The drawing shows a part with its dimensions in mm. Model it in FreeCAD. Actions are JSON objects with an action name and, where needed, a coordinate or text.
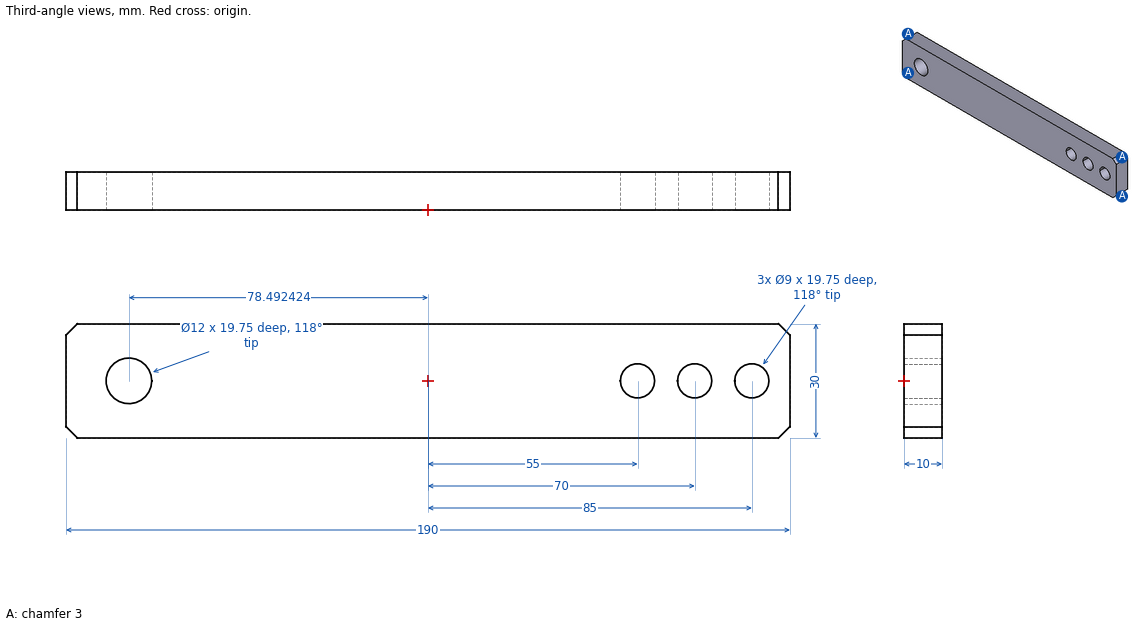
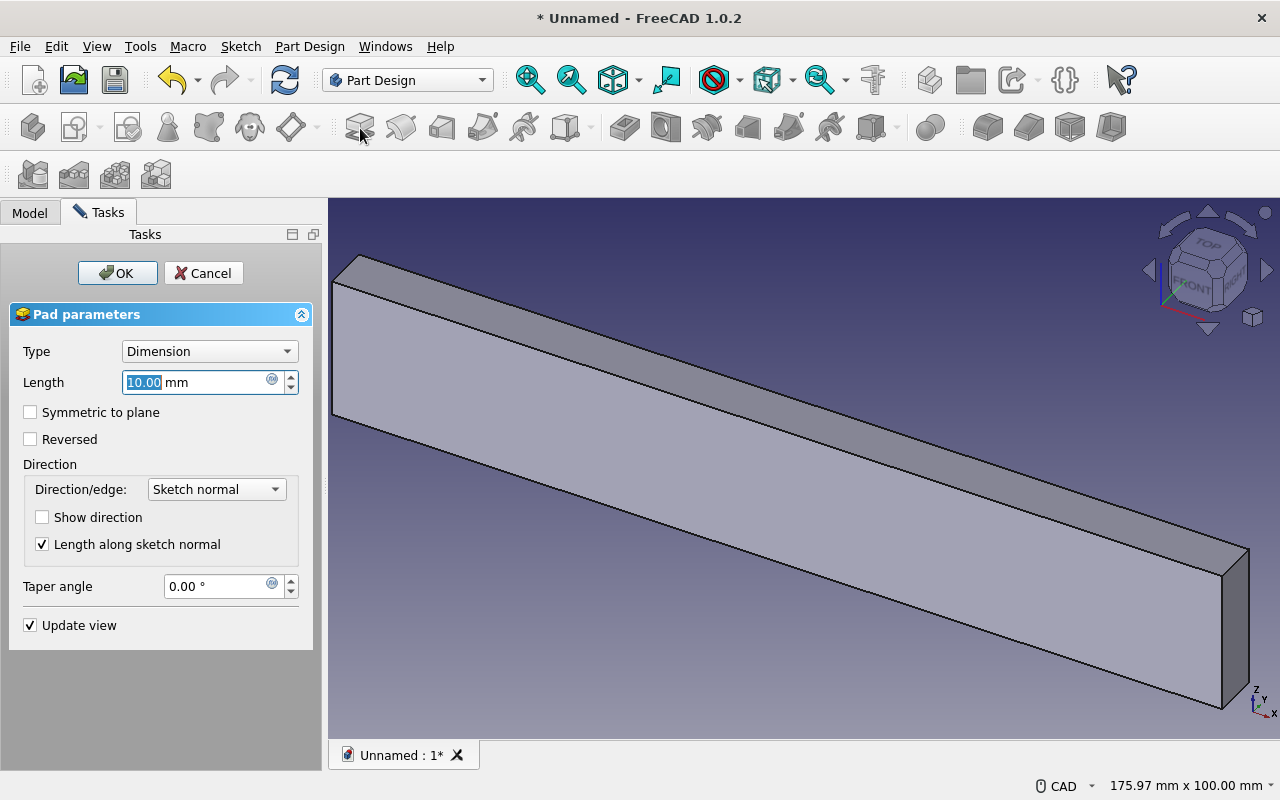
{"action": "type", "text": "10"}
{"action": "key", "text": "Tab"}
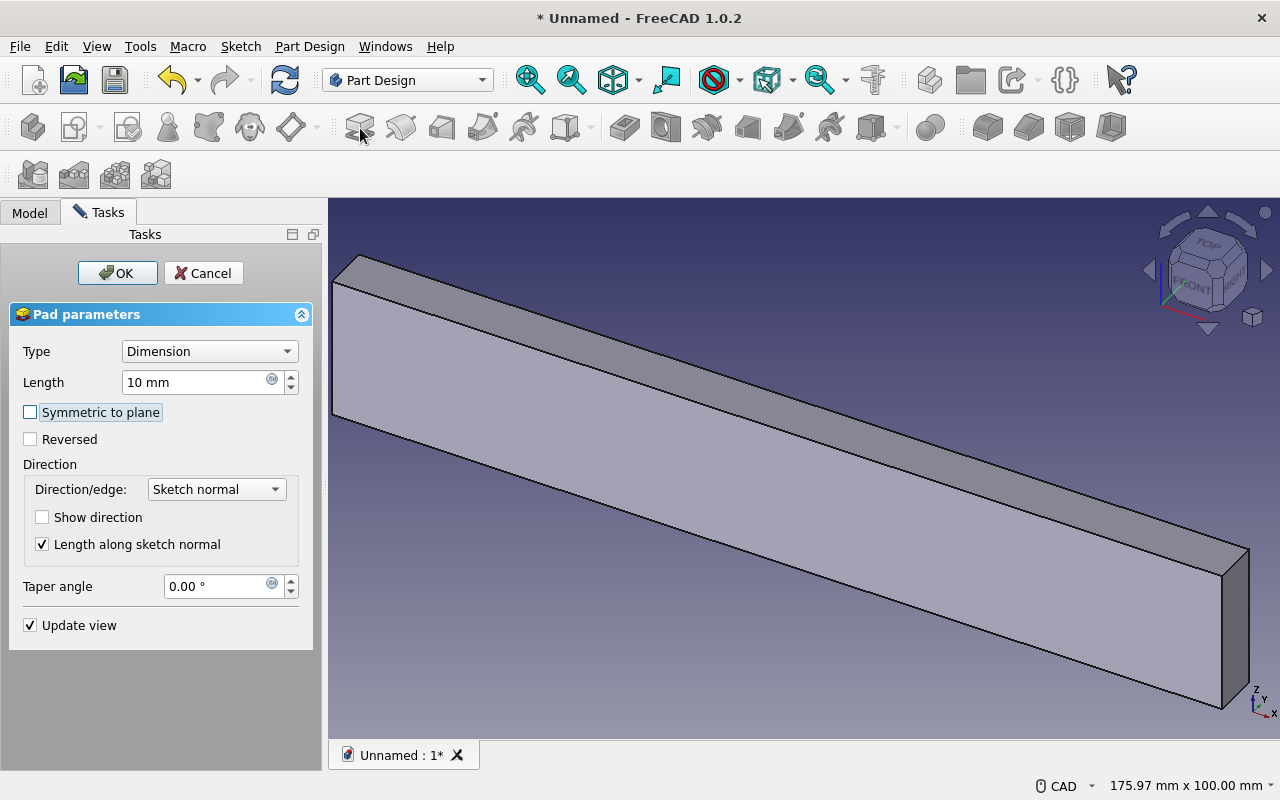
{"action": "left_click", "coordinate": [31, 439]}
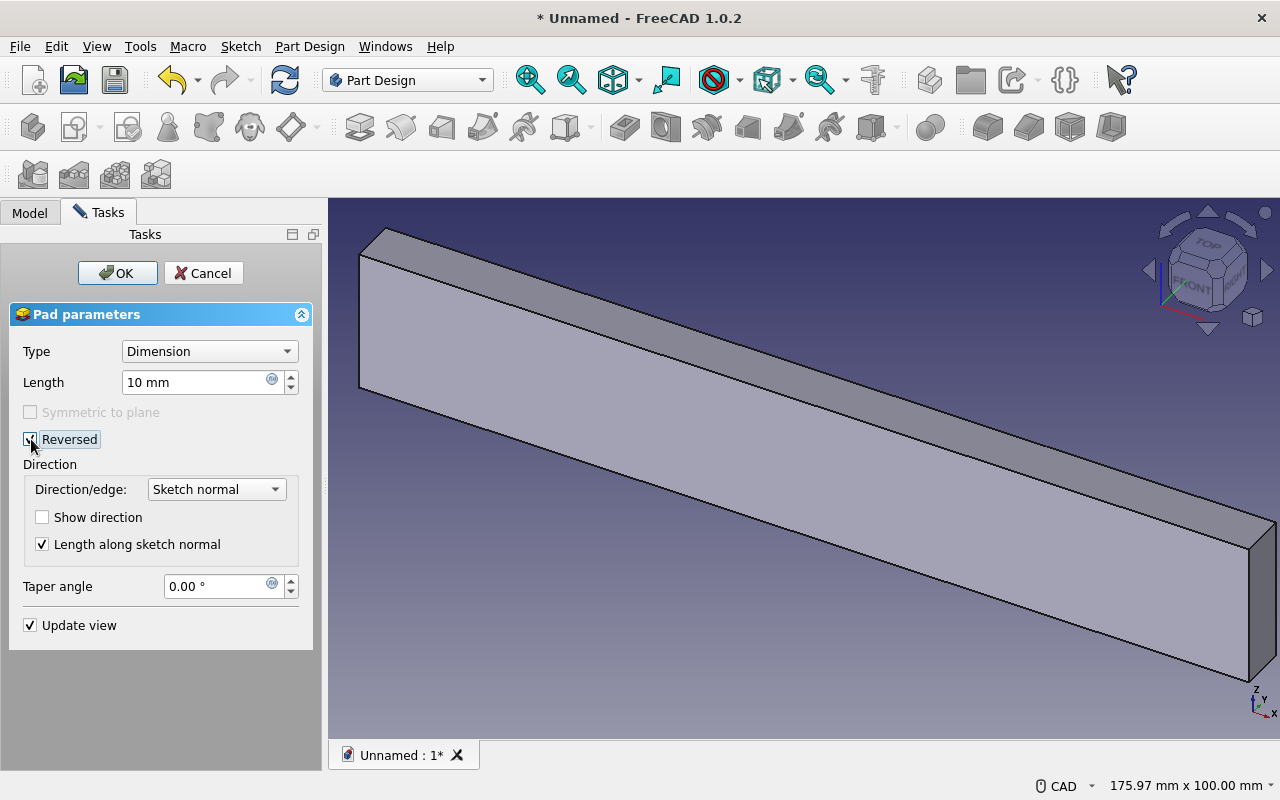
{"action": "left_click", "coordinate": [118, 273]}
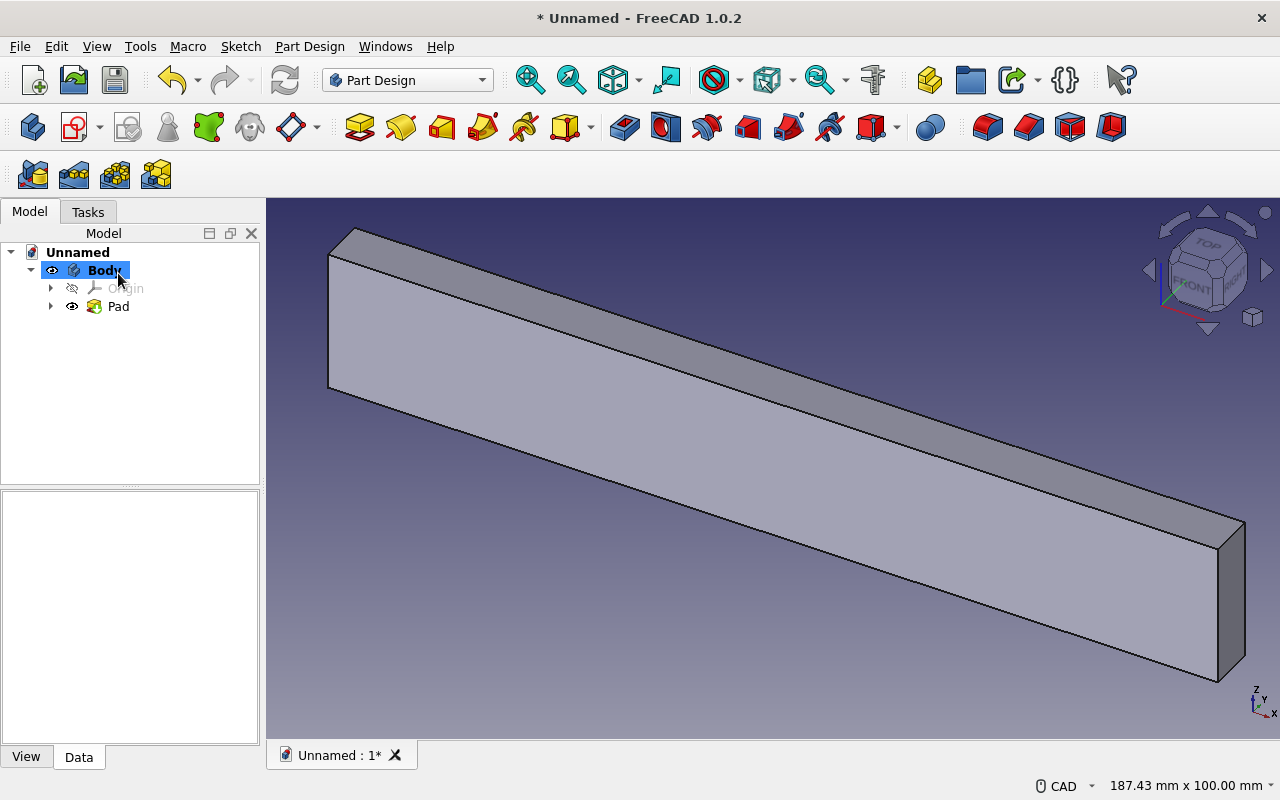
{"action": "key", "text": "0"}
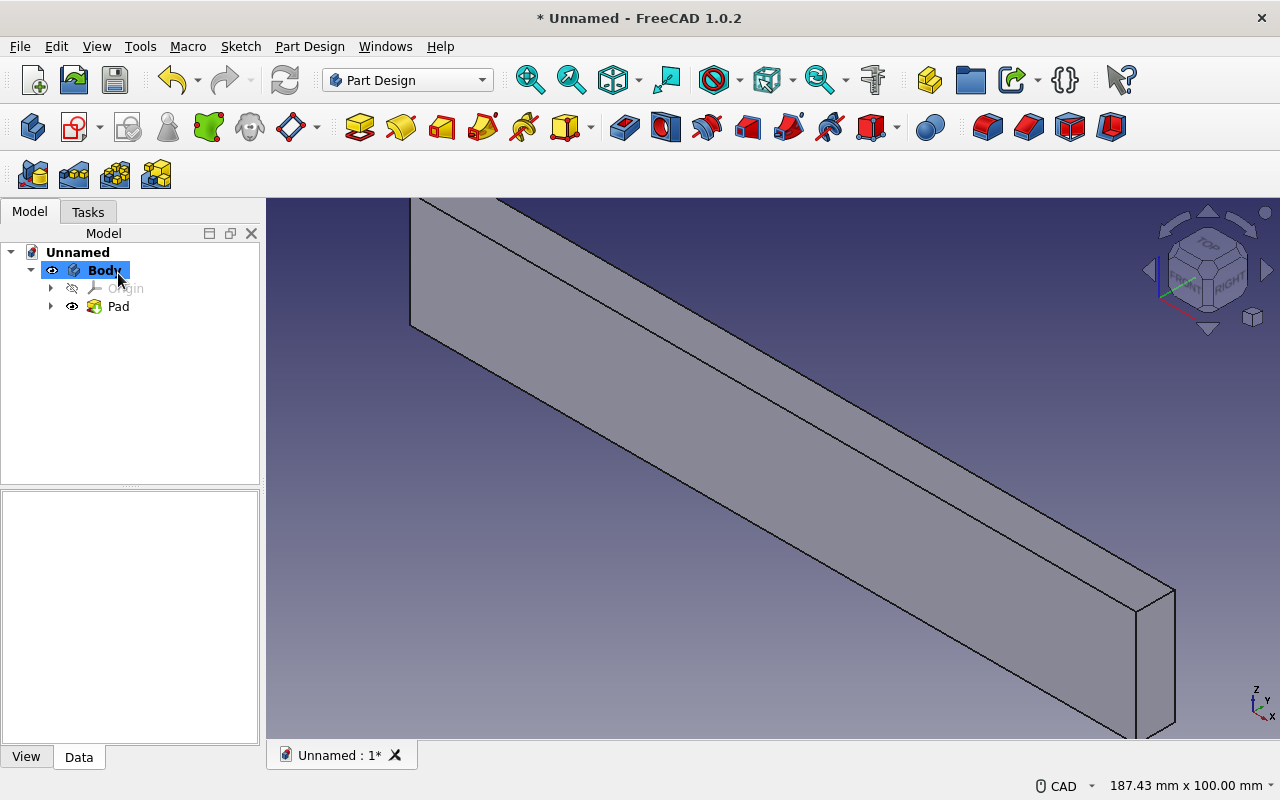
{"action": "key", "text": "v f"}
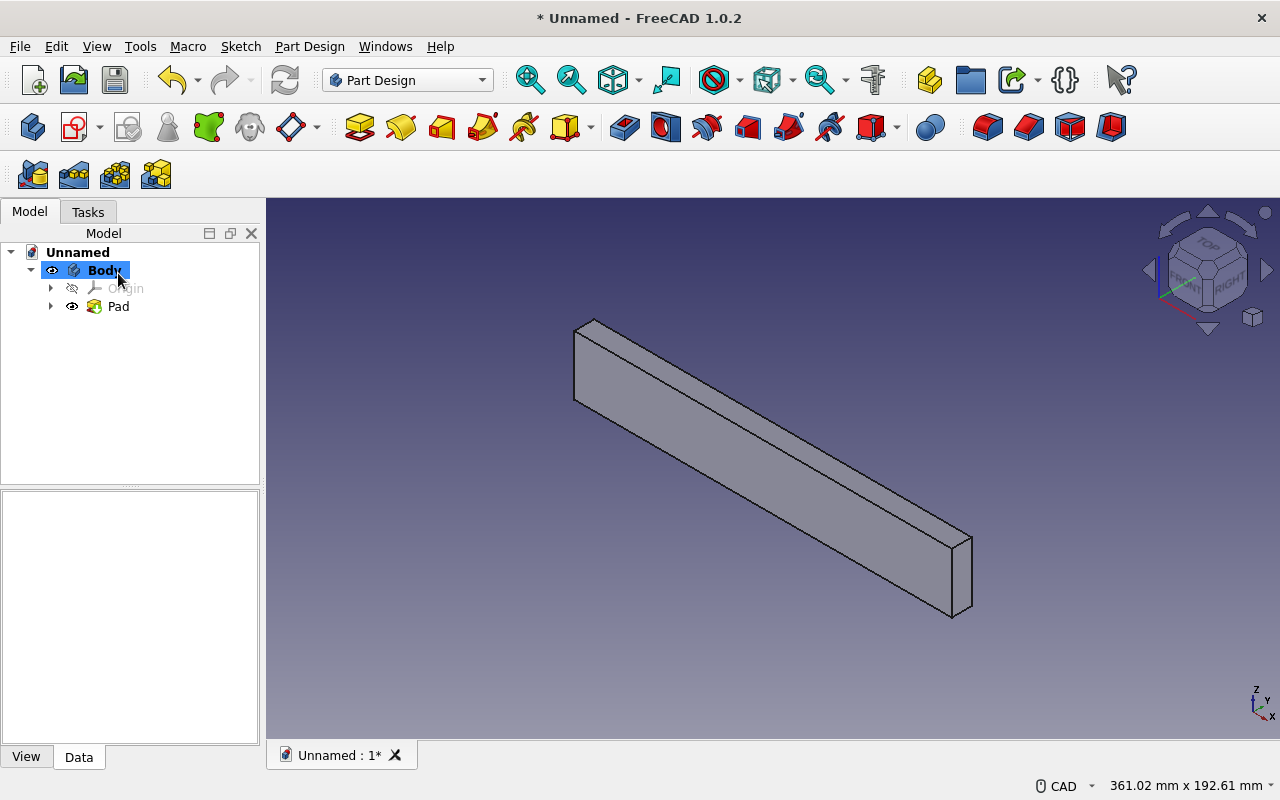
{"action": "left_click", "coordinate": [962, 542]}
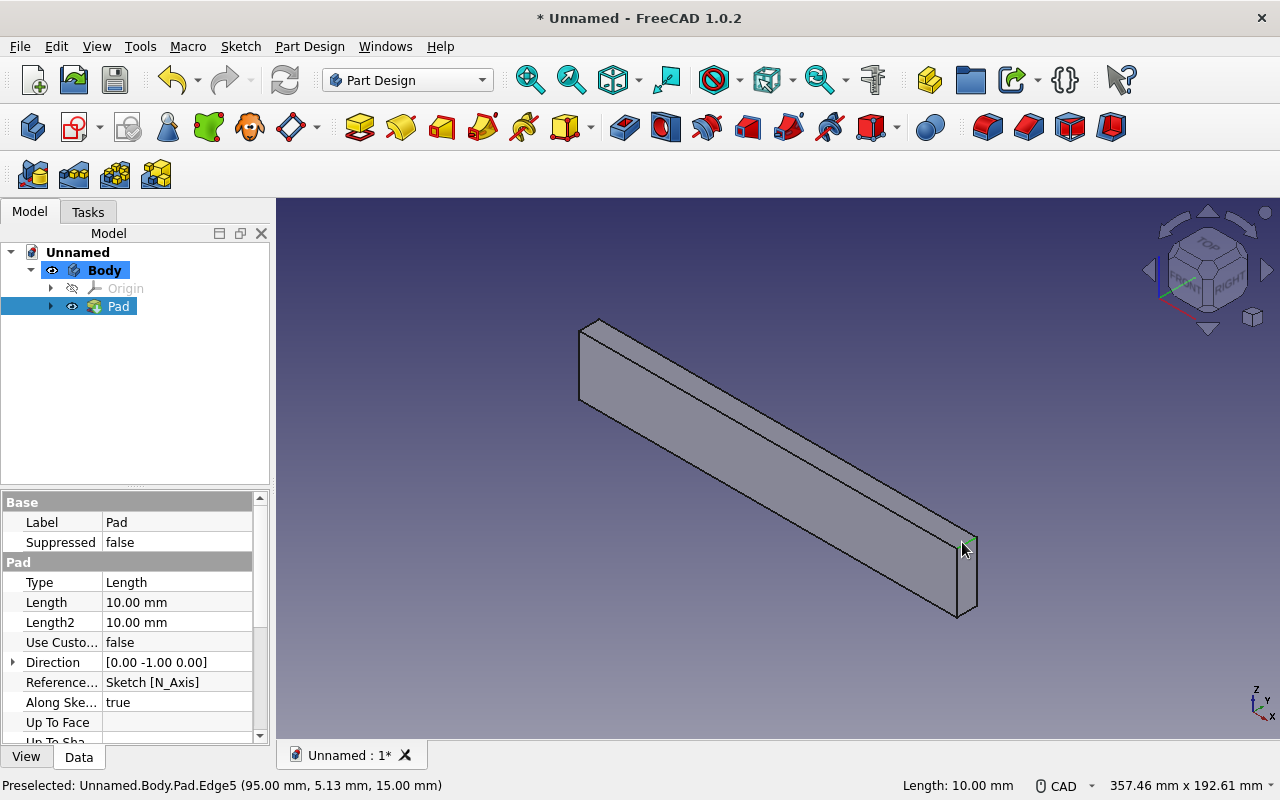
{"action": "key", "text": "2"}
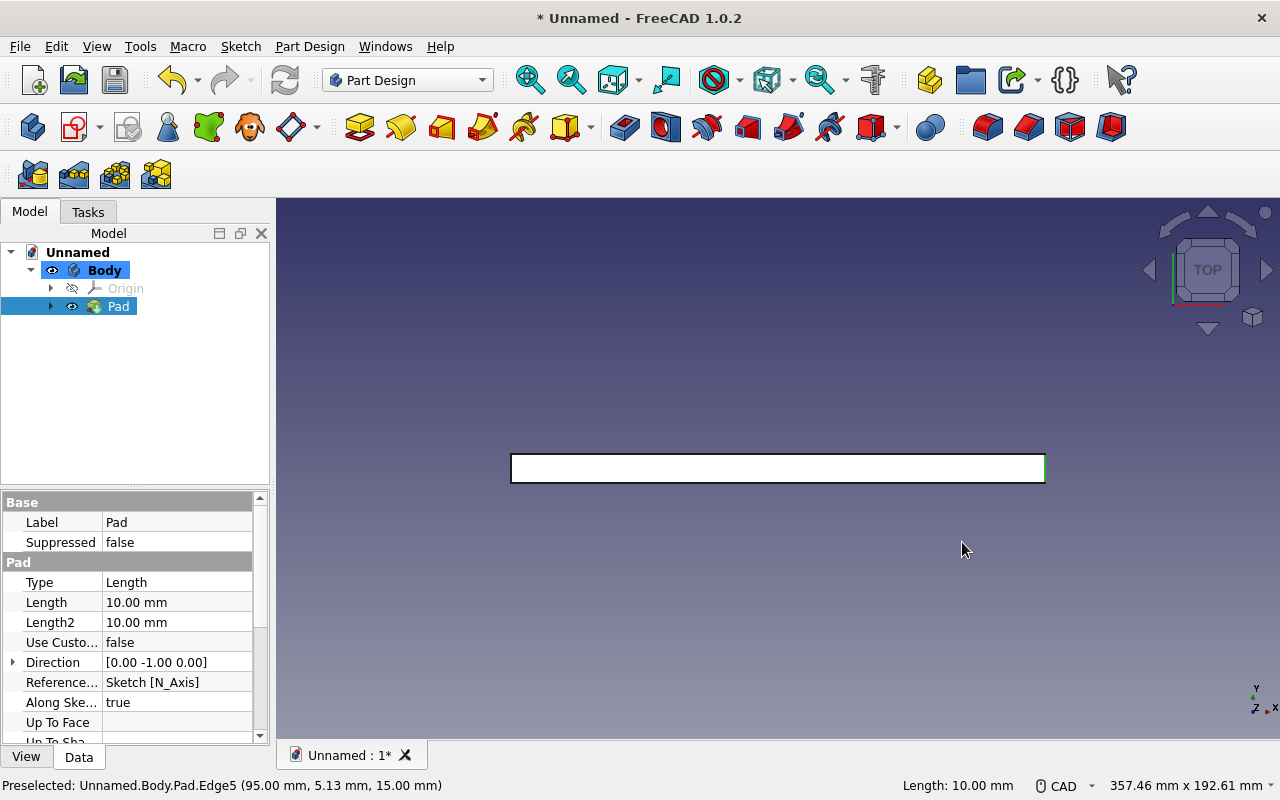
{"action": "left_click", "coordinate": [511, 467], "text": "ctrl"}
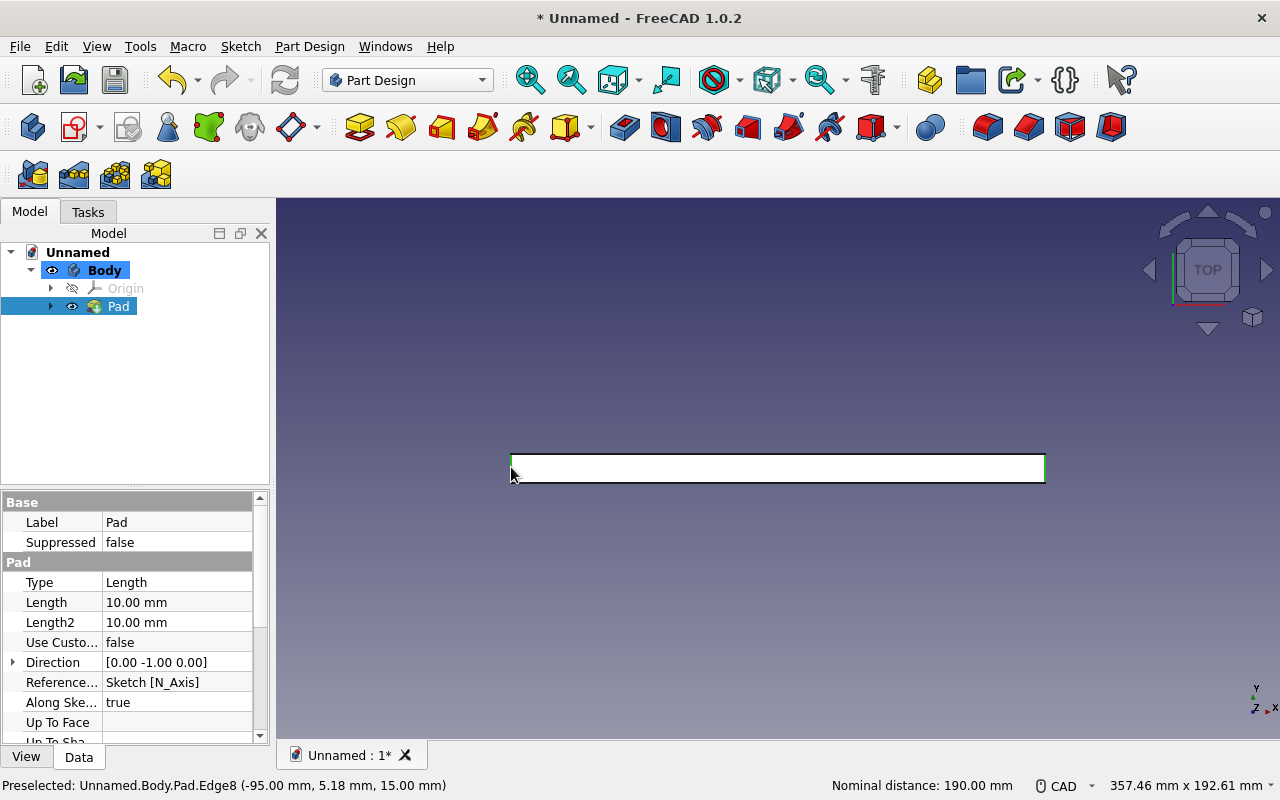
{"action": "key", "text": "1"}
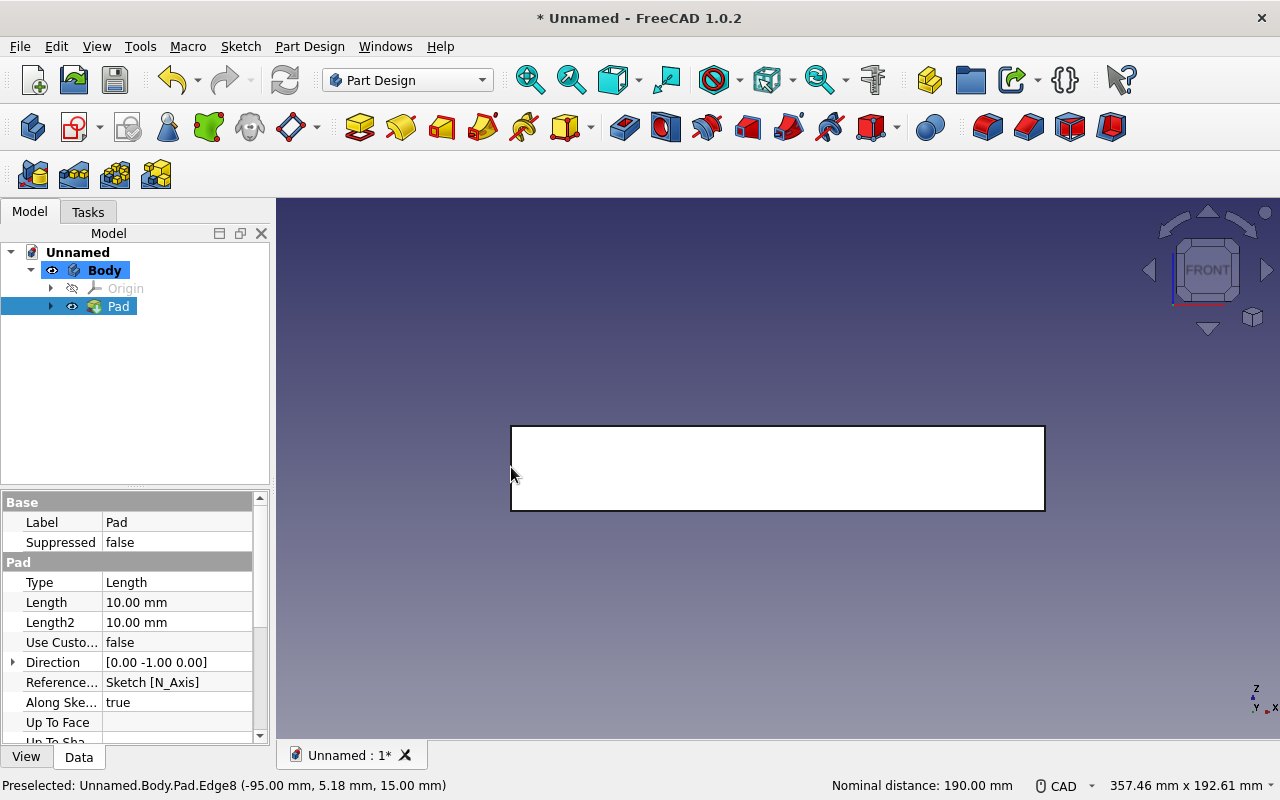
{"action": "key", "text": "3"}